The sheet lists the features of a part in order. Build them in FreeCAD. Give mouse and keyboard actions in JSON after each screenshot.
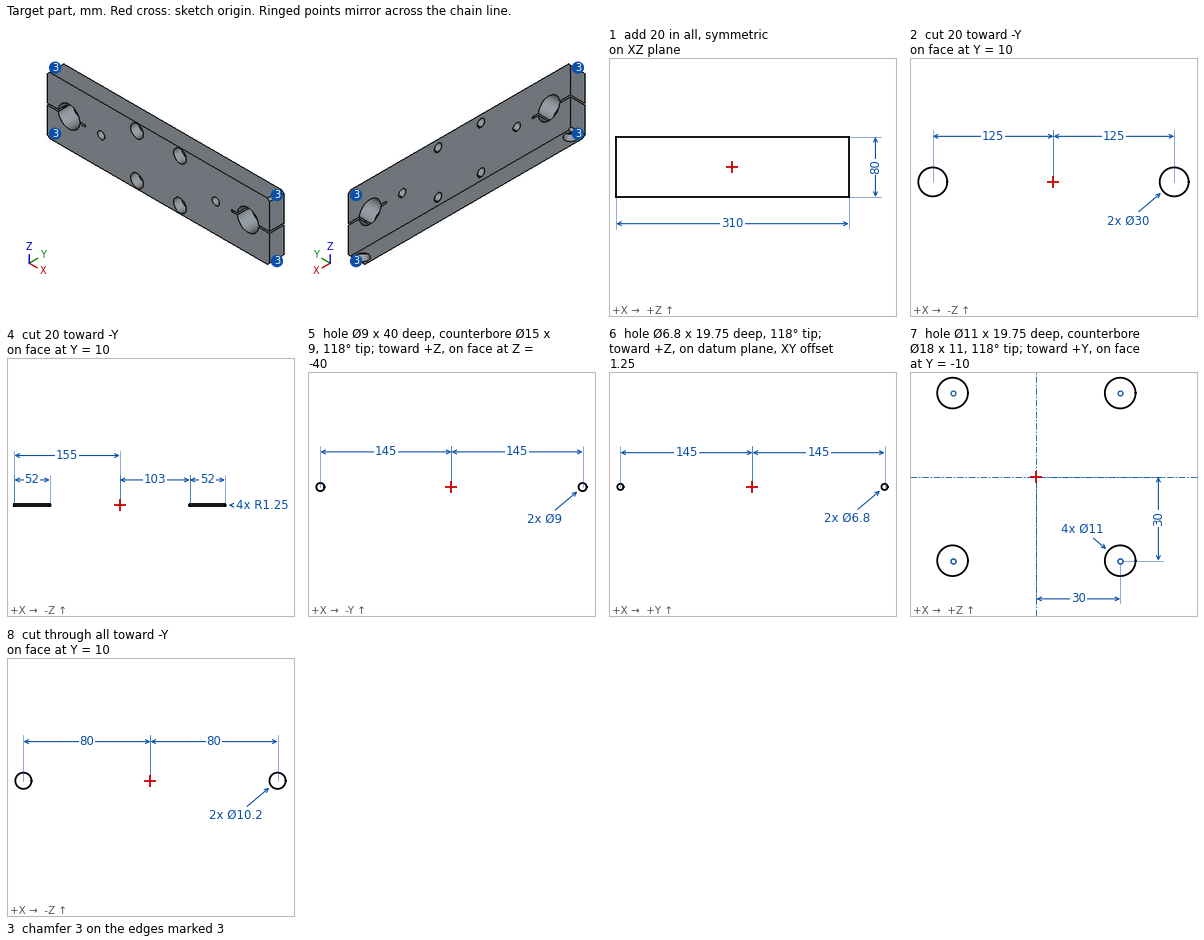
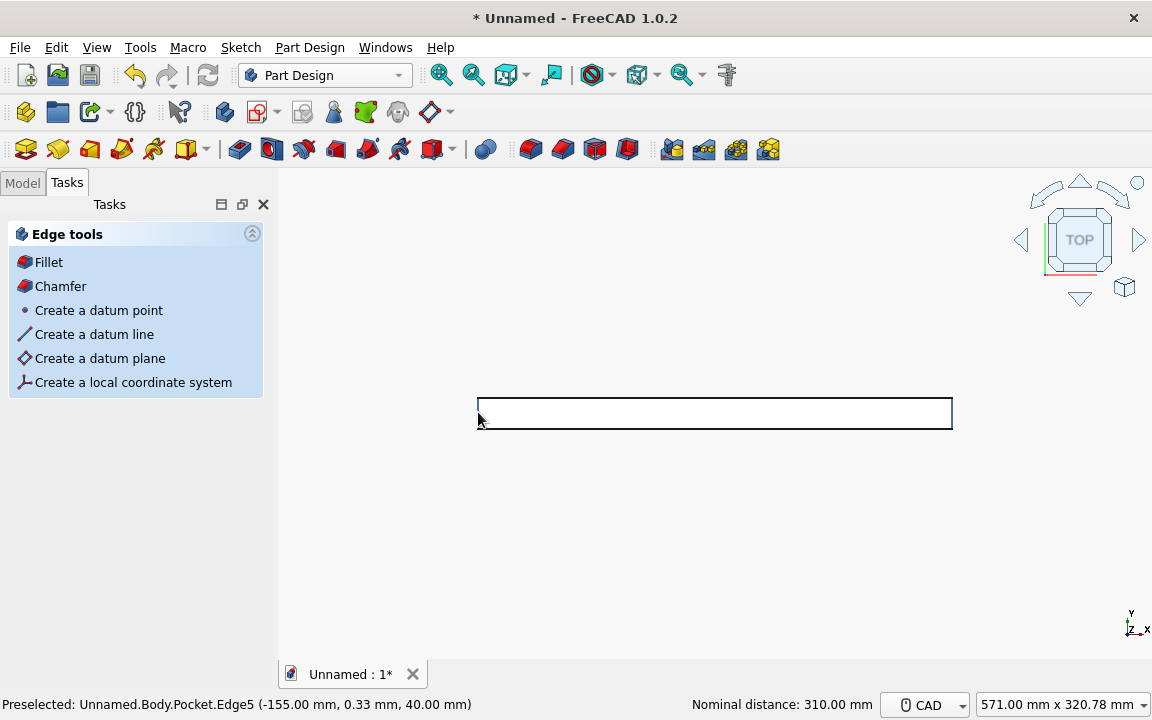
{"action": "key", "text": "1"}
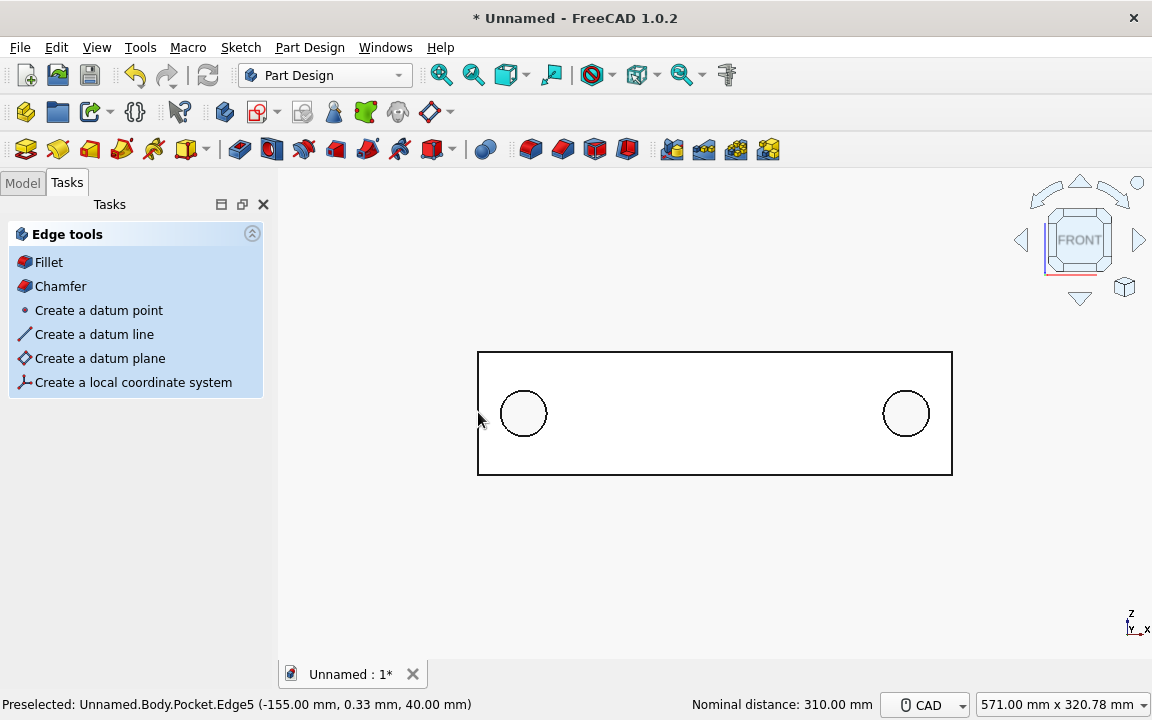
{"action": "key", "text": "3"}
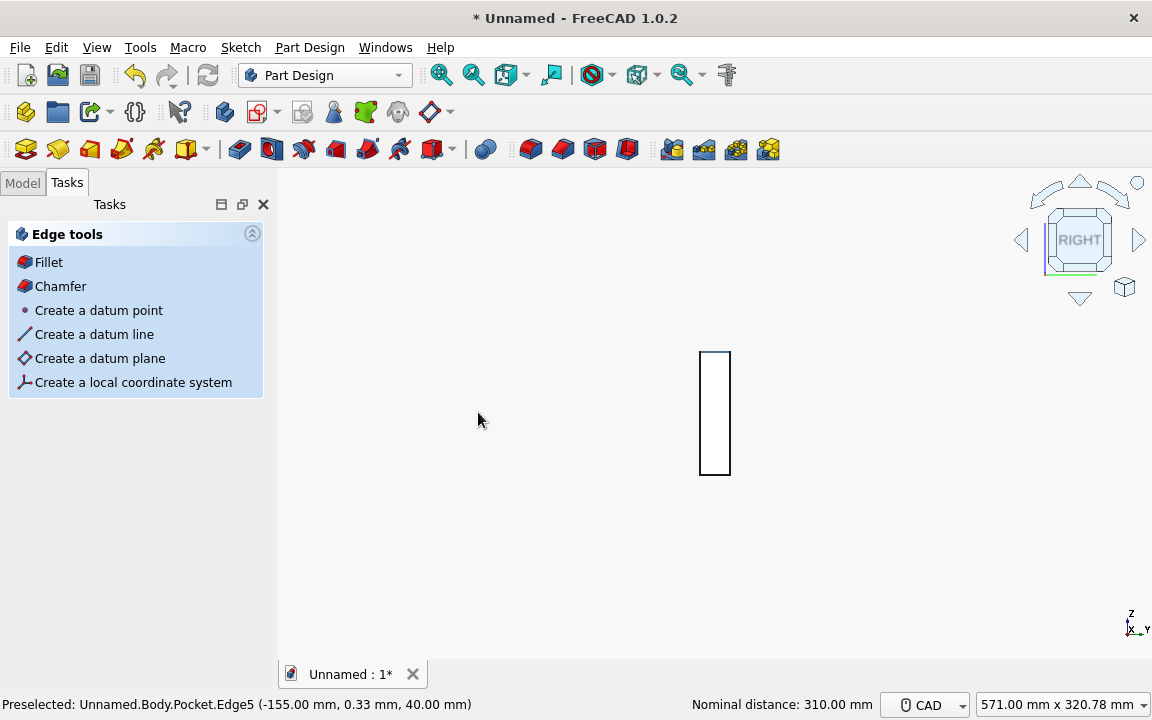
{"action": "left_click", "coordinate": [442, 76]}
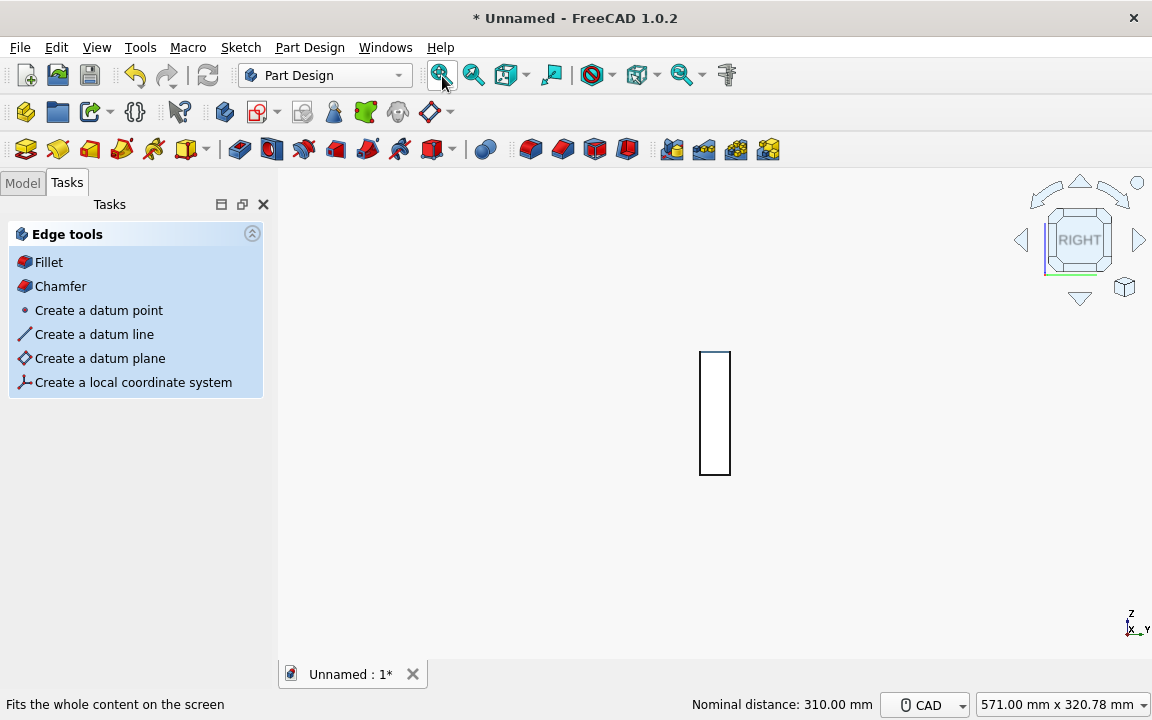
{"action": "left_click", "coordinate": [715, 474], "text": "ctrl"}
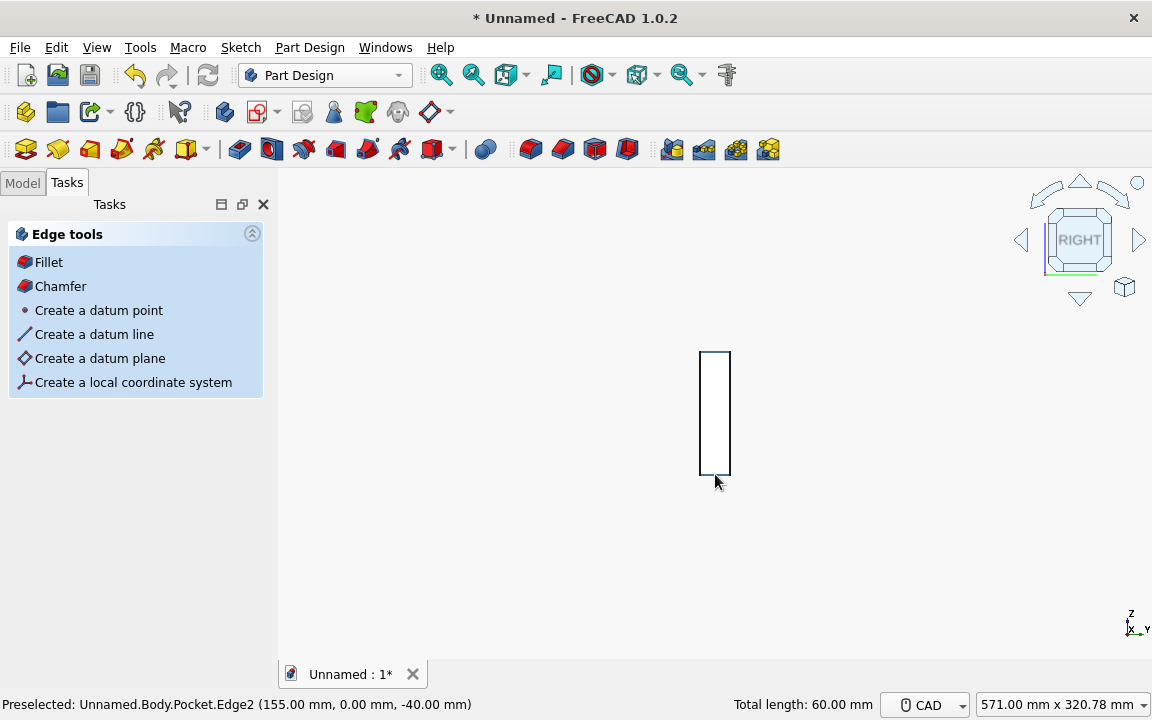
{"action": "key", "text": "5"}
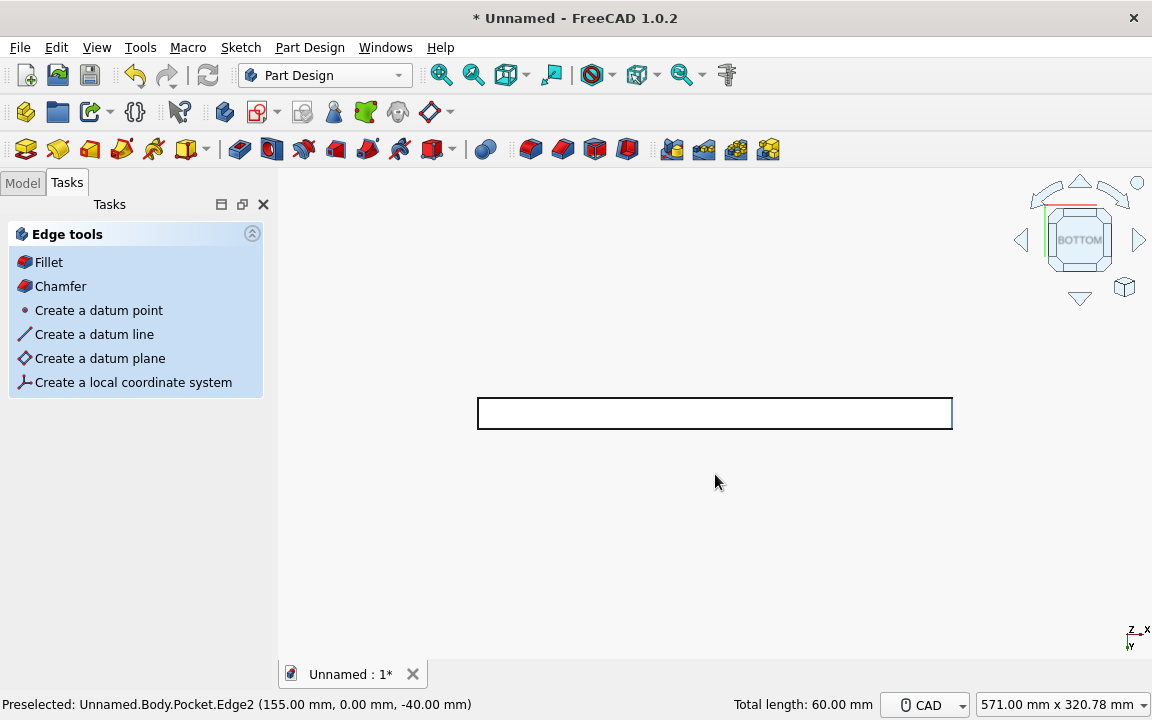
{"action": "left_click", "coordinate": [478, 412], "text": "ctrl"}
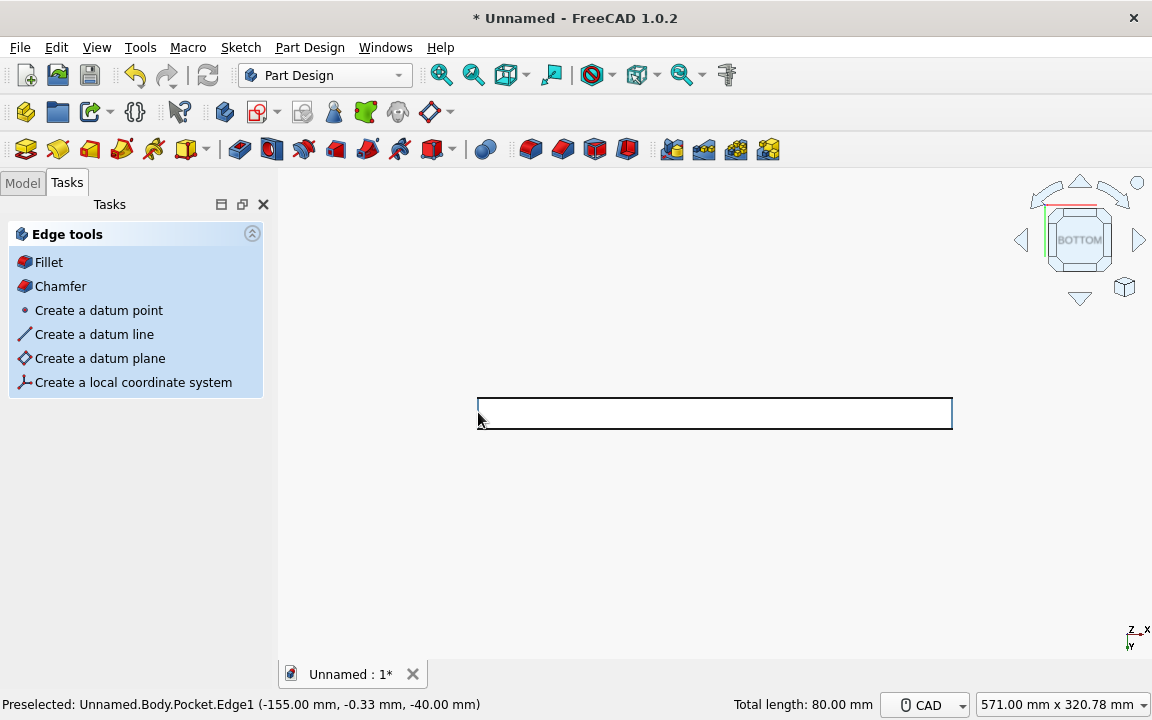
{"action": "left_click", "coordinate": [564, 150]}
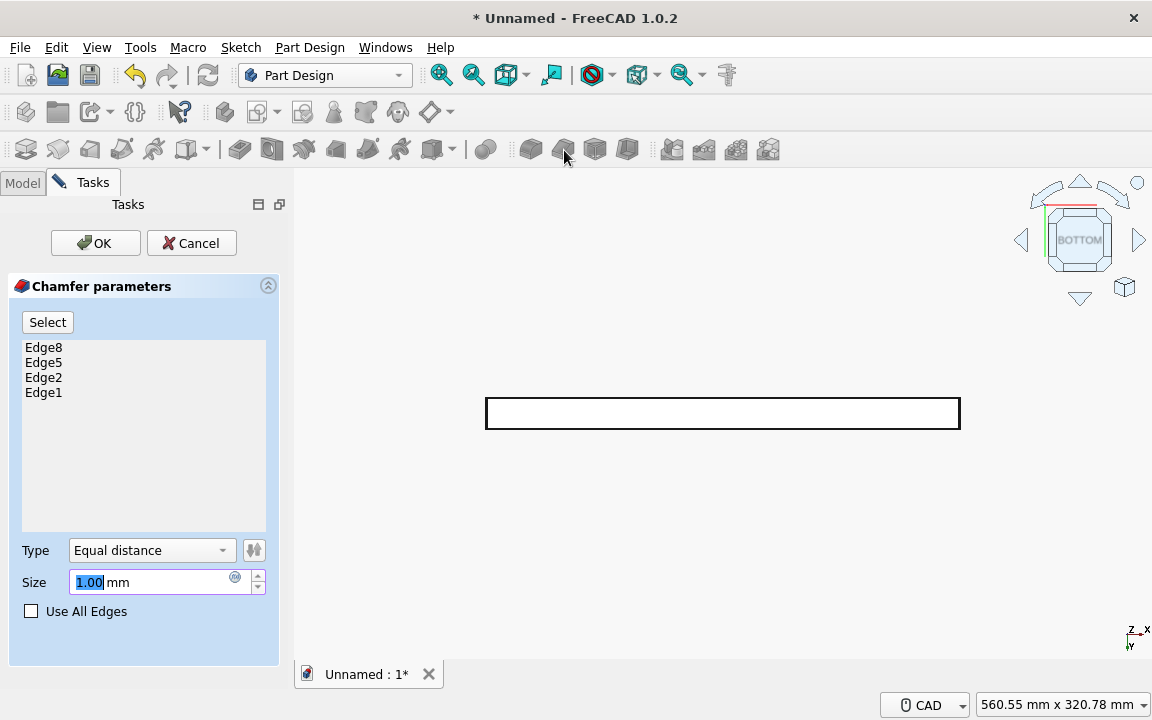
{"action": "type", "text": "3"}
{"action": "key", "text": "Tab"}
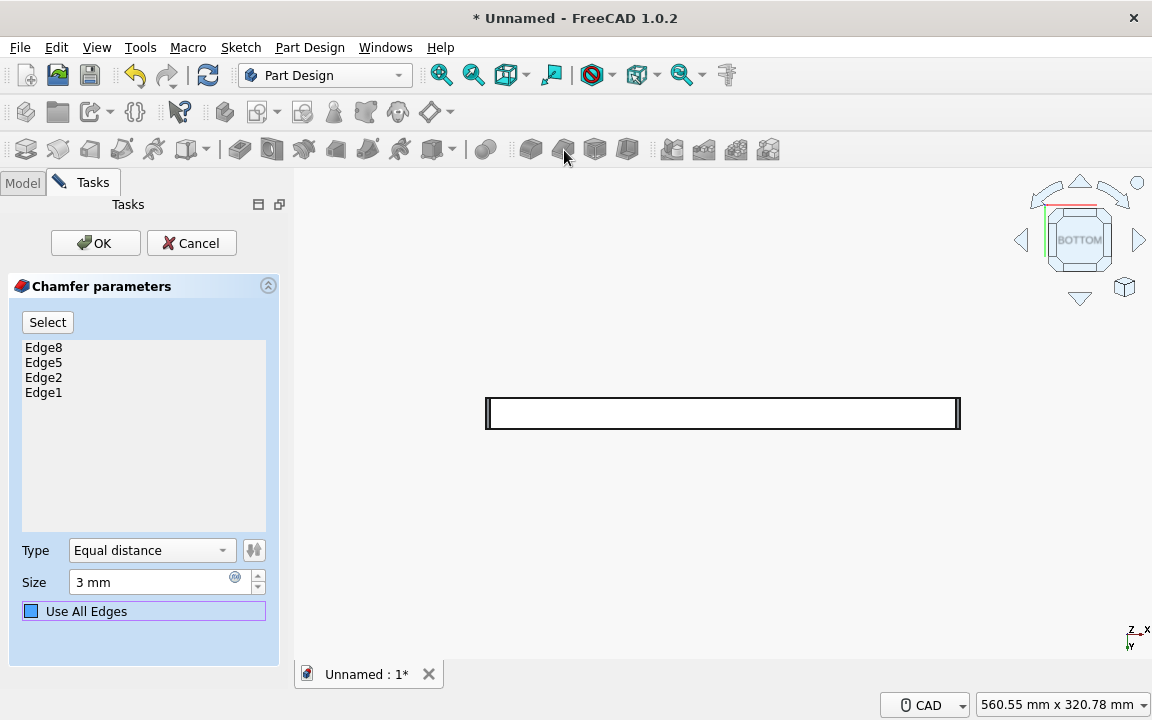
{"action": "left_click", "coordinate": [96, 243]}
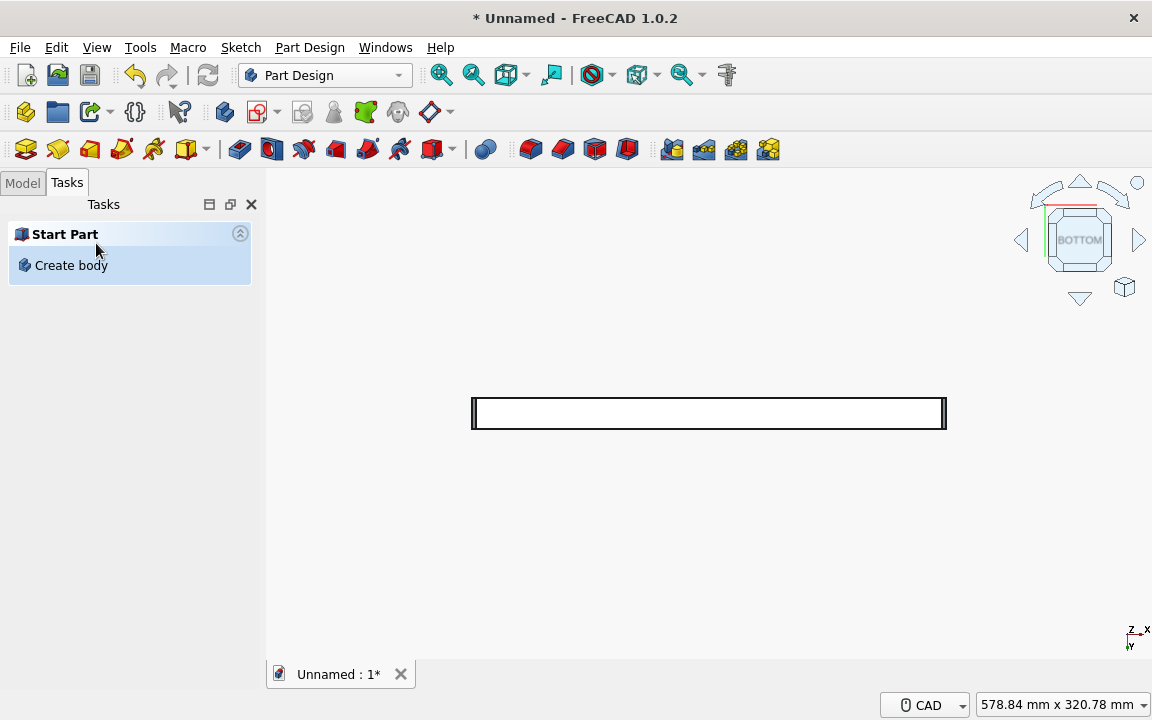
{"action": "key", "text": "4"}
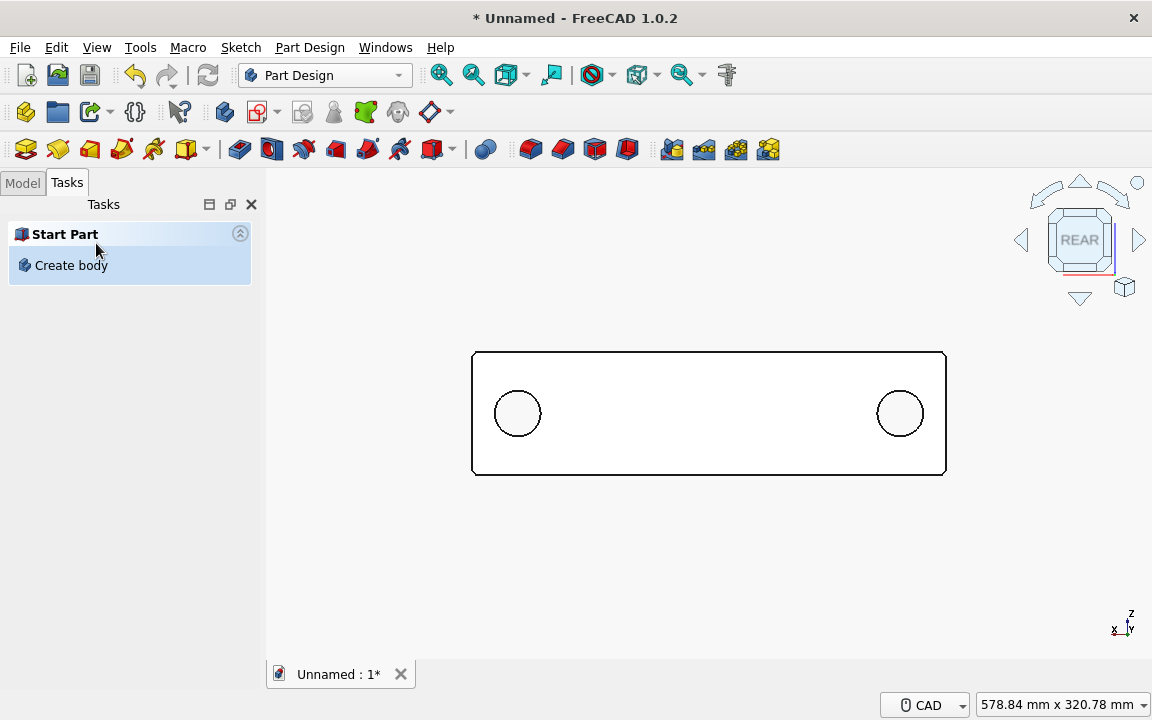
{"action": "left_click", "coordinate": [641, 412]}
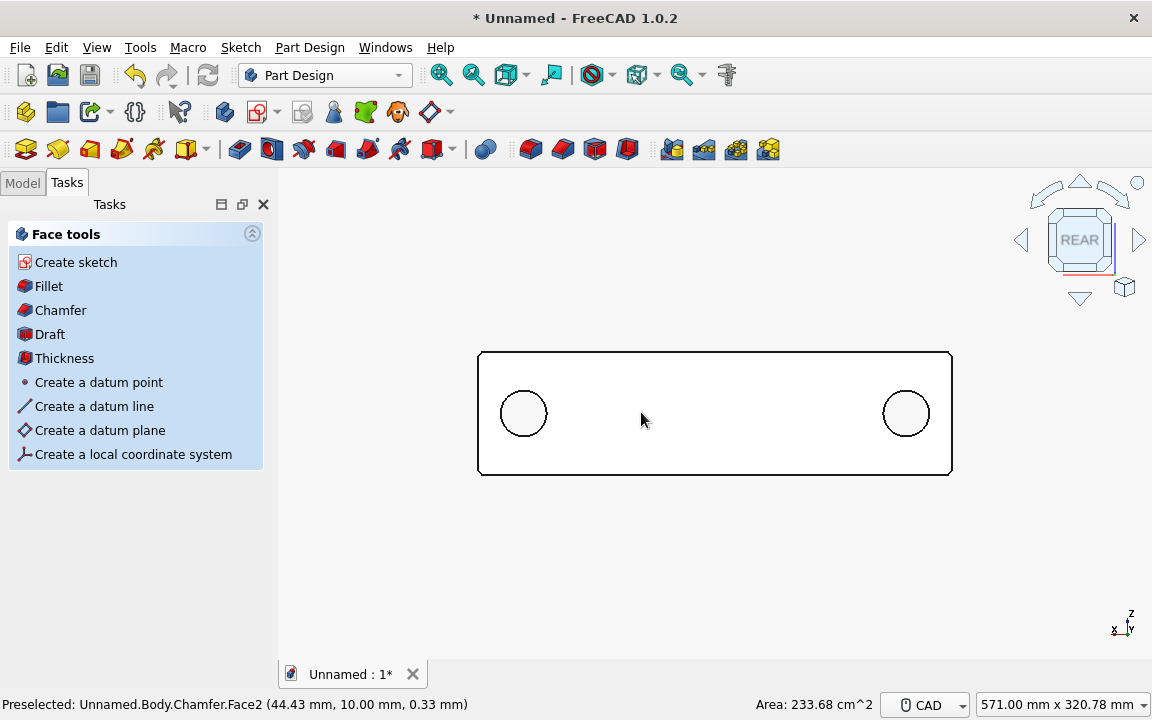
{"action": "left_click", "coordinate": [258, 112]}